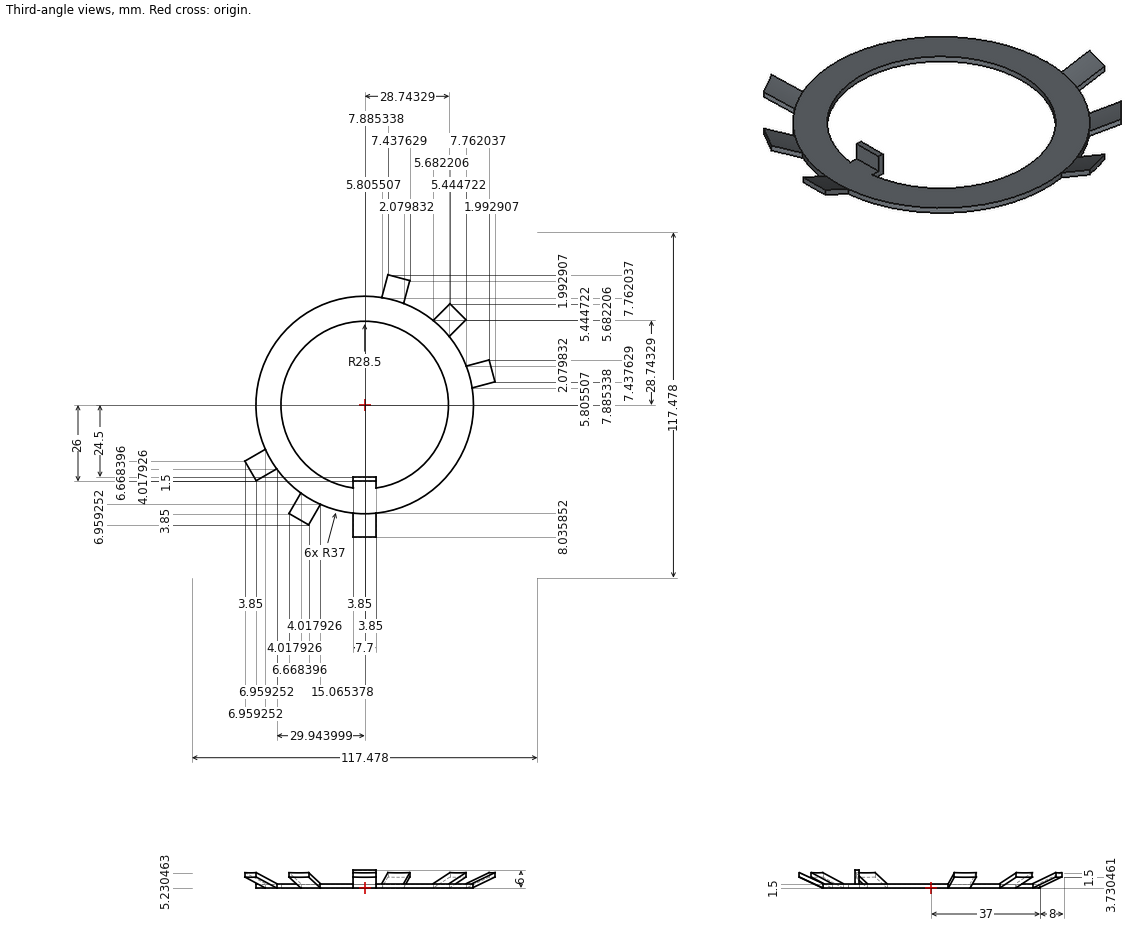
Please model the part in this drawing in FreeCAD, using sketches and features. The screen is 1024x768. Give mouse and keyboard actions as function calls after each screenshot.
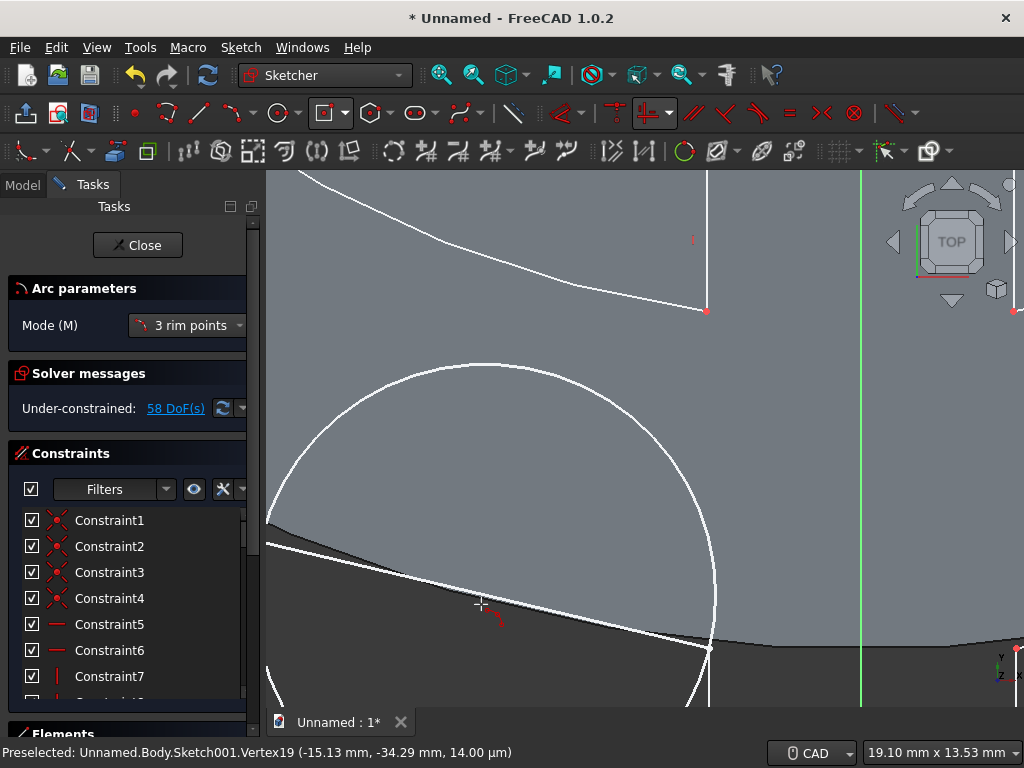
click(481, 599)
key(Escape)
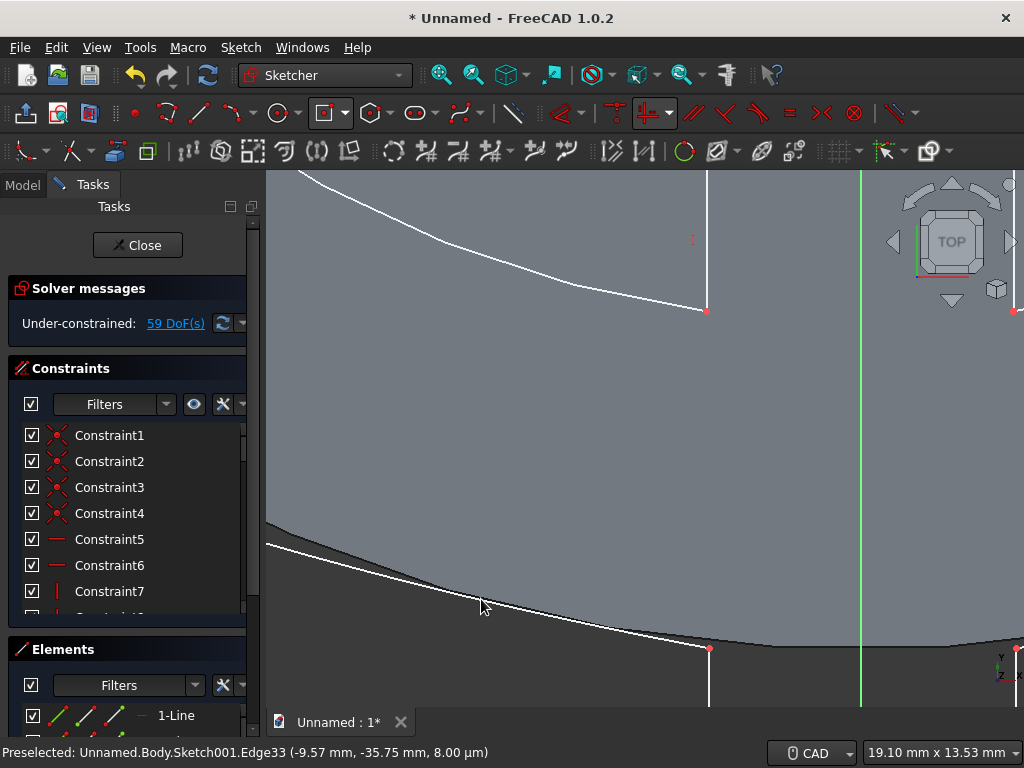
scroll(554, 539, down, 13)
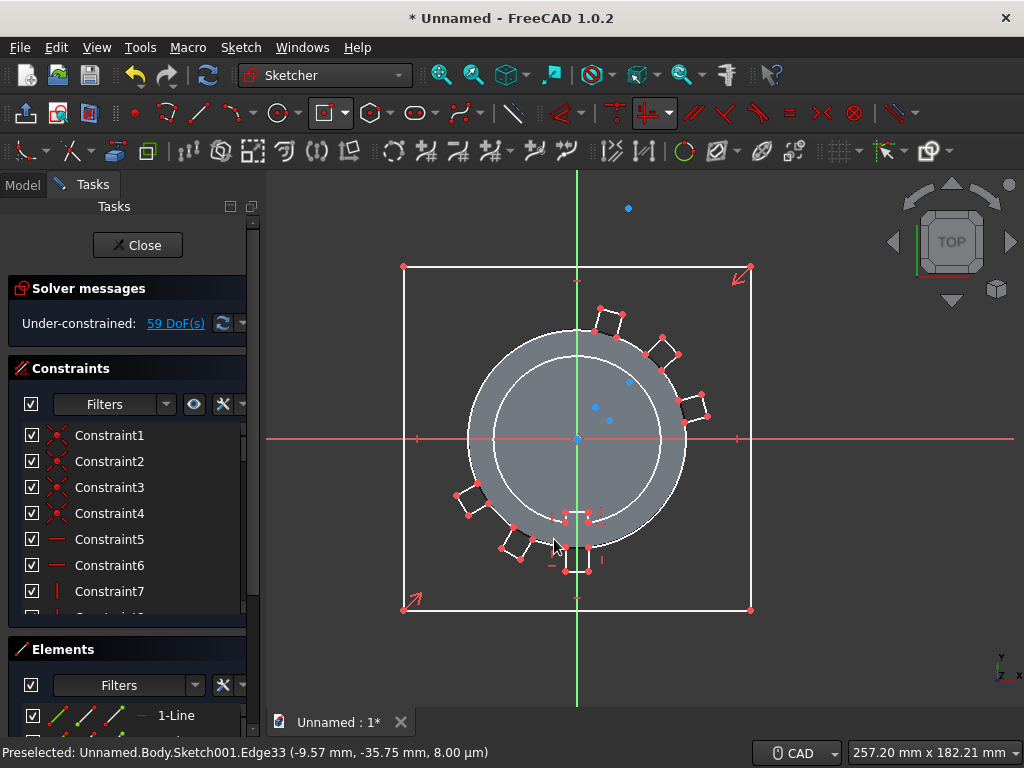
click(655, 410)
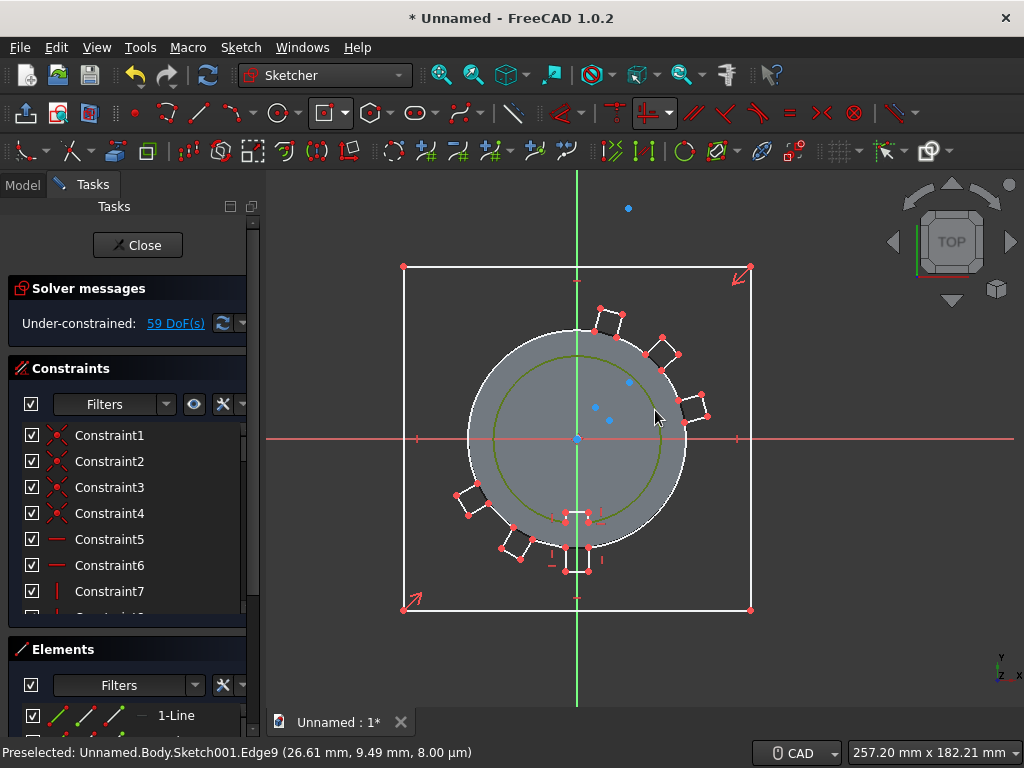
scroll(496, 512, up, 2)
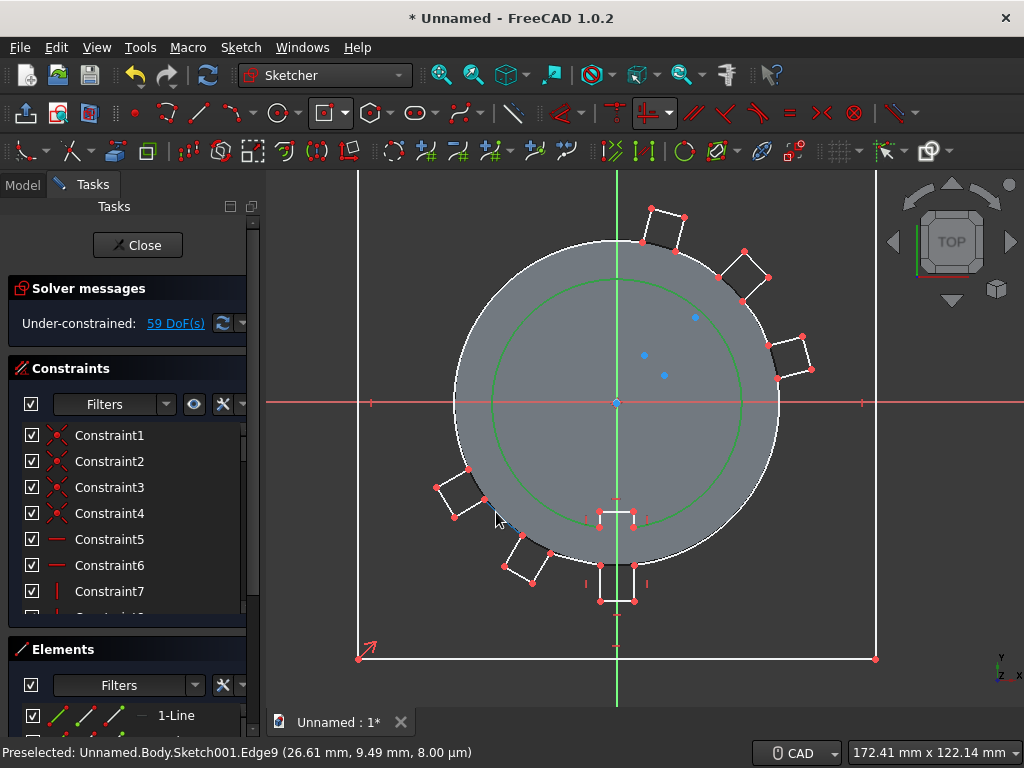
click(495, 511)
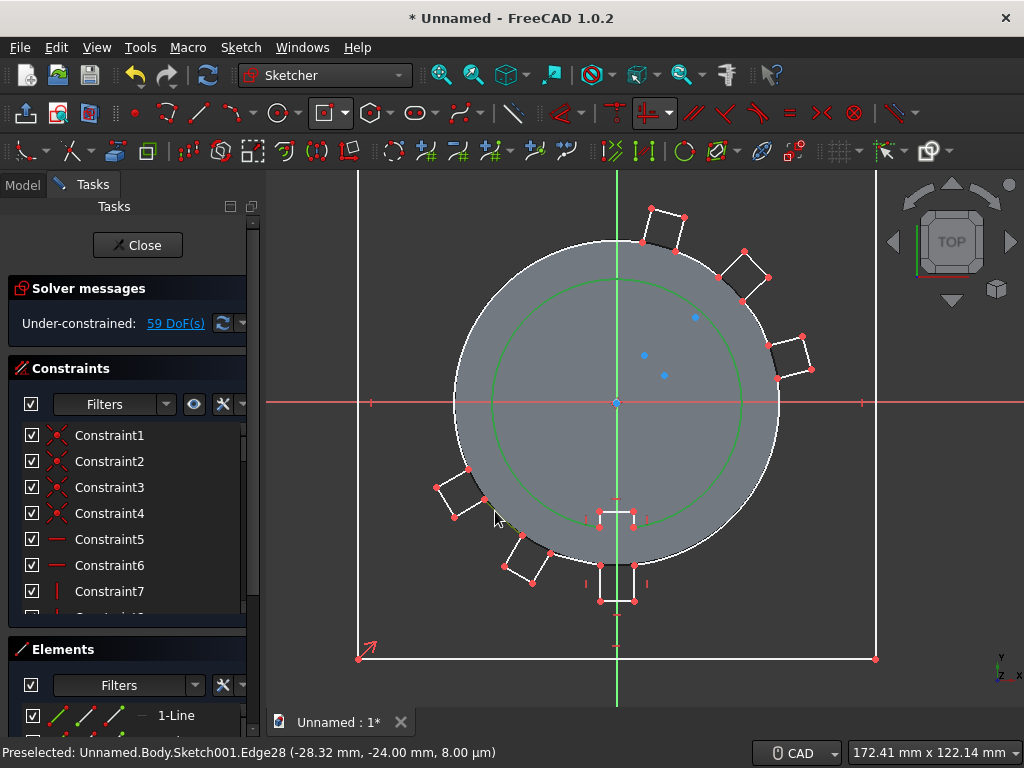
key(c)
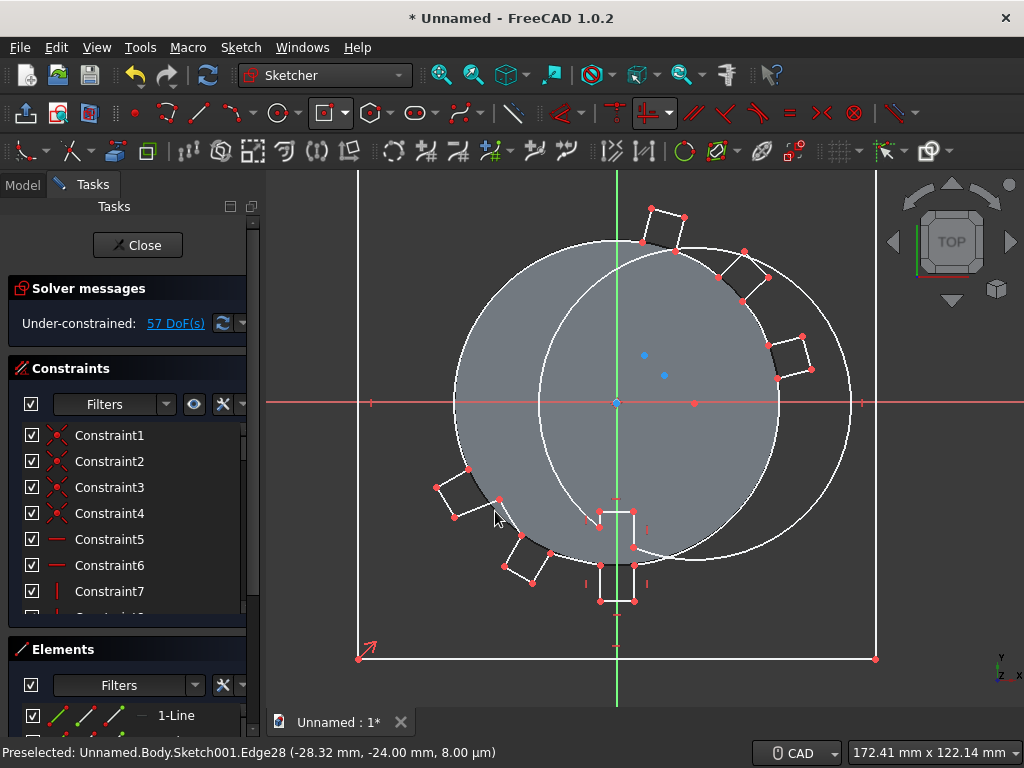
click(849, 429)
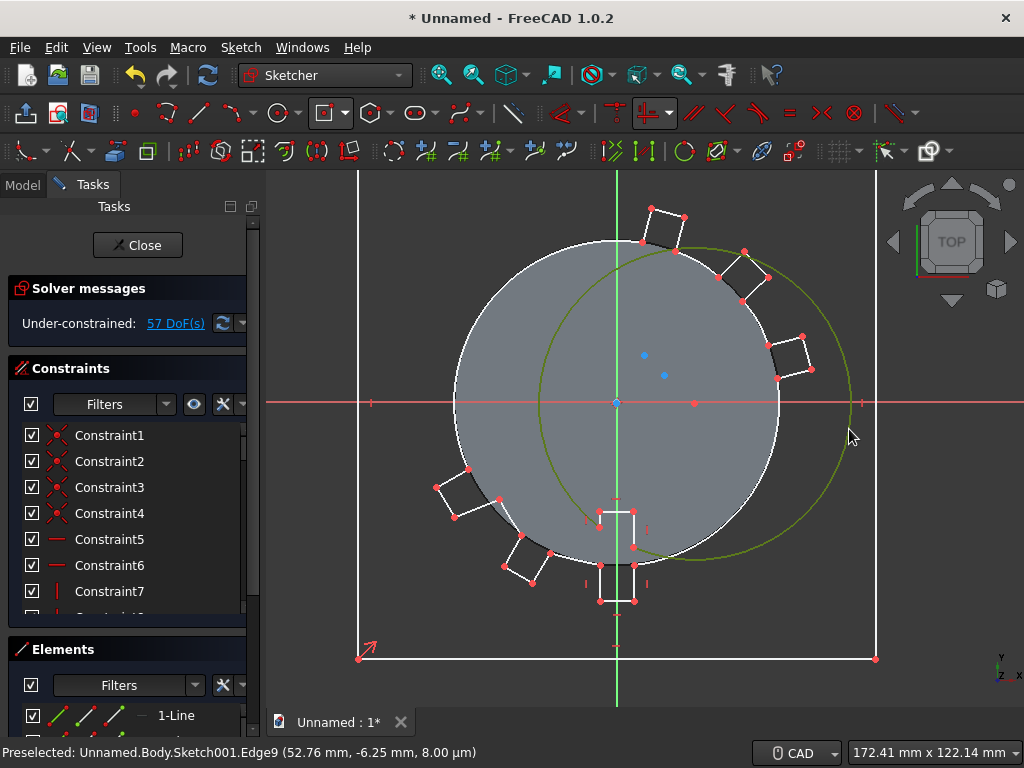
click(541, 259)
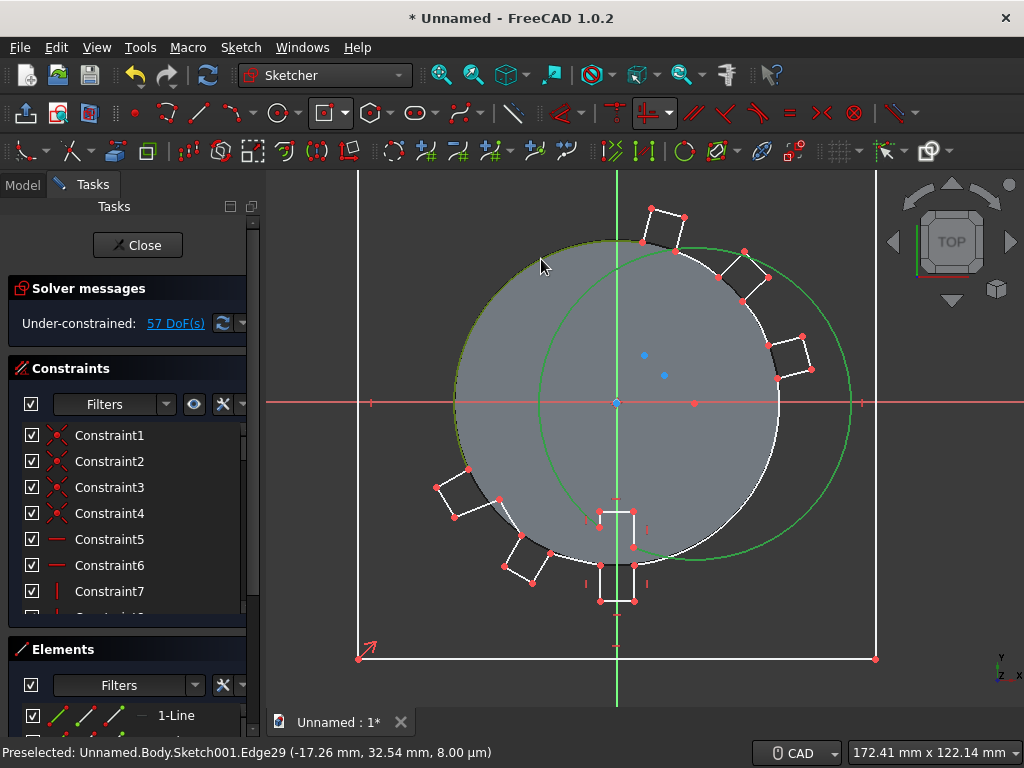
click(616, 114)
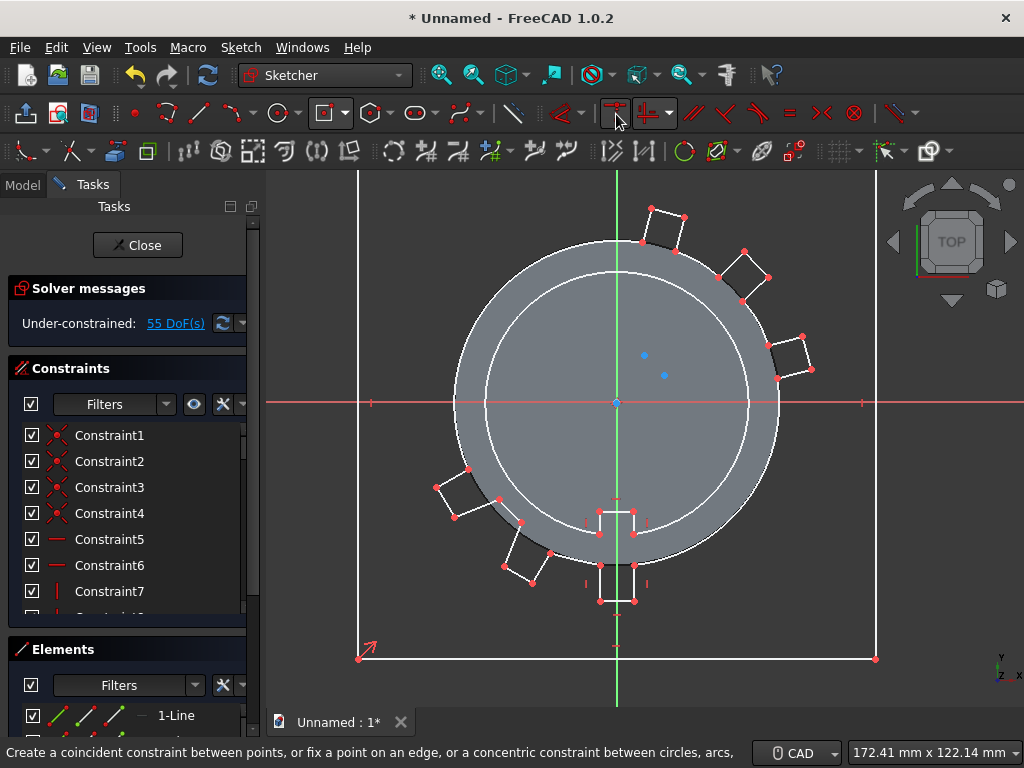
click(740, 357)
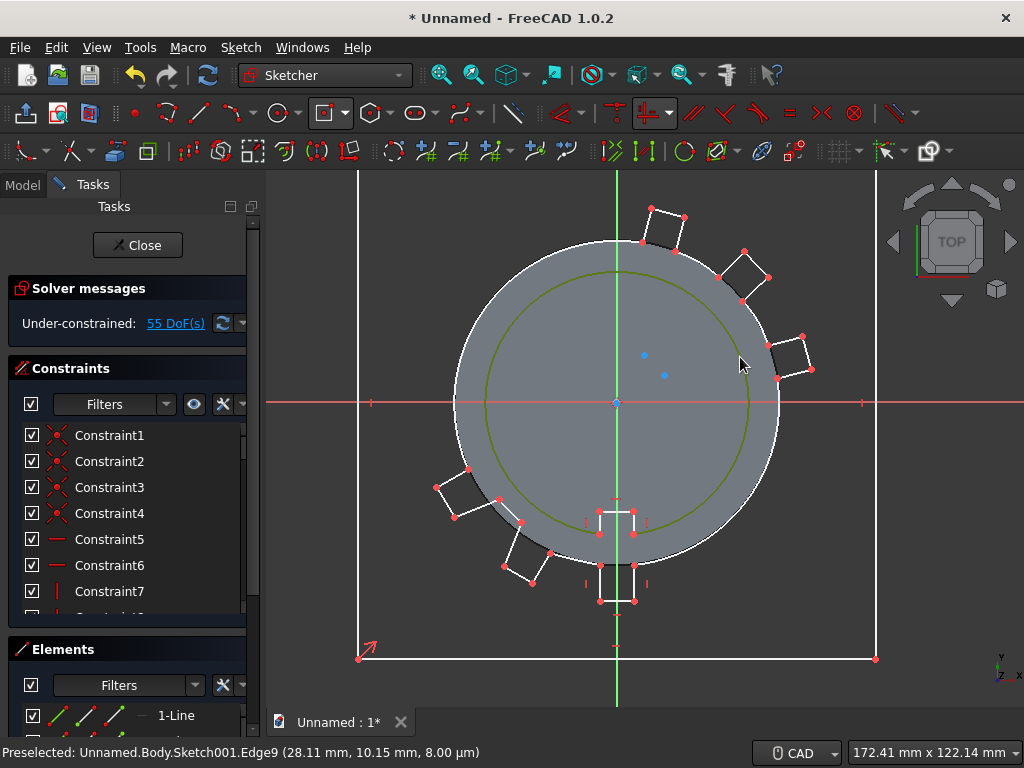
click(707, 268)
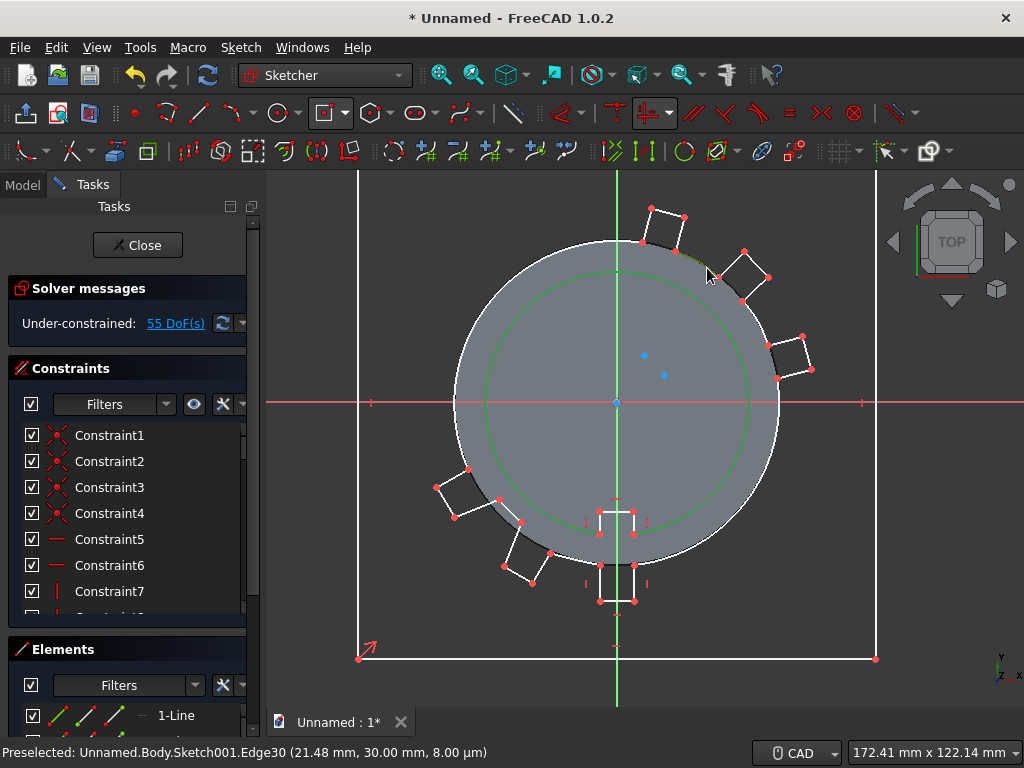
click(616, 114)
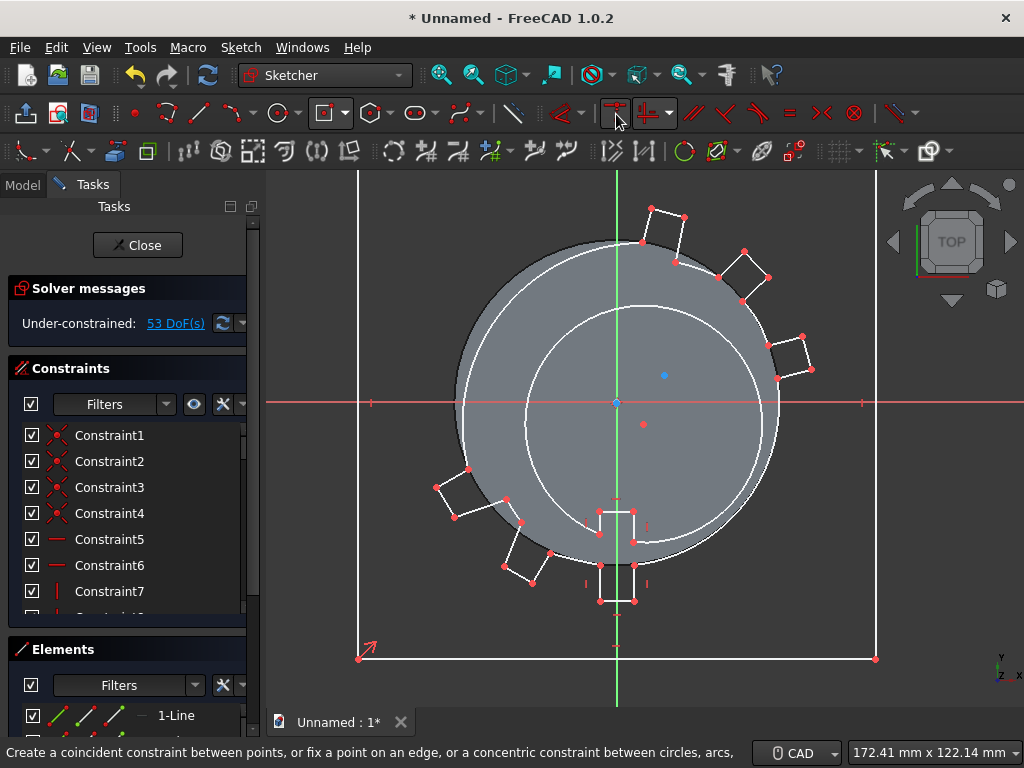
click(546, 357)